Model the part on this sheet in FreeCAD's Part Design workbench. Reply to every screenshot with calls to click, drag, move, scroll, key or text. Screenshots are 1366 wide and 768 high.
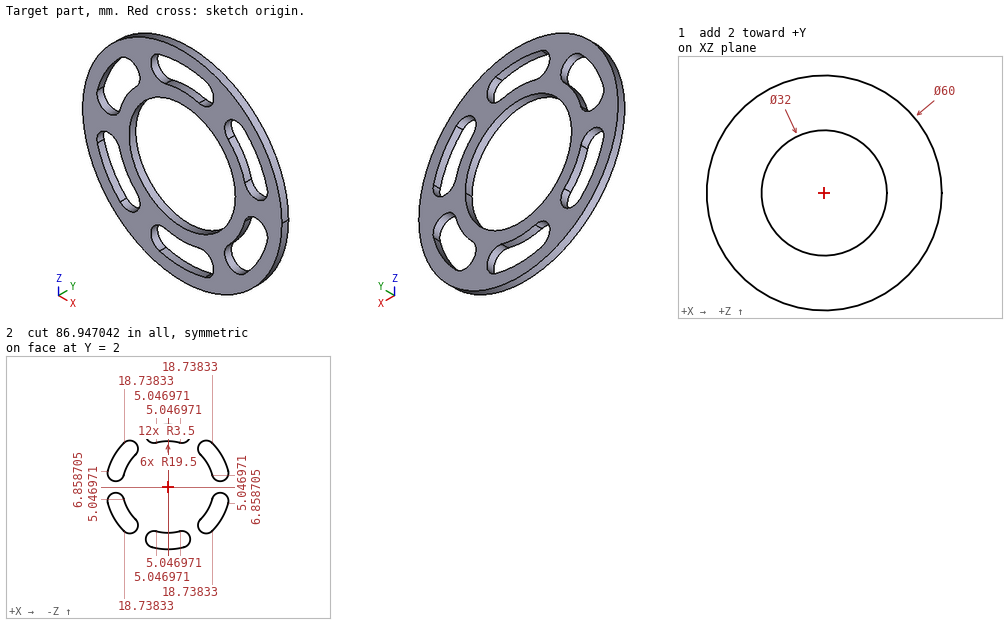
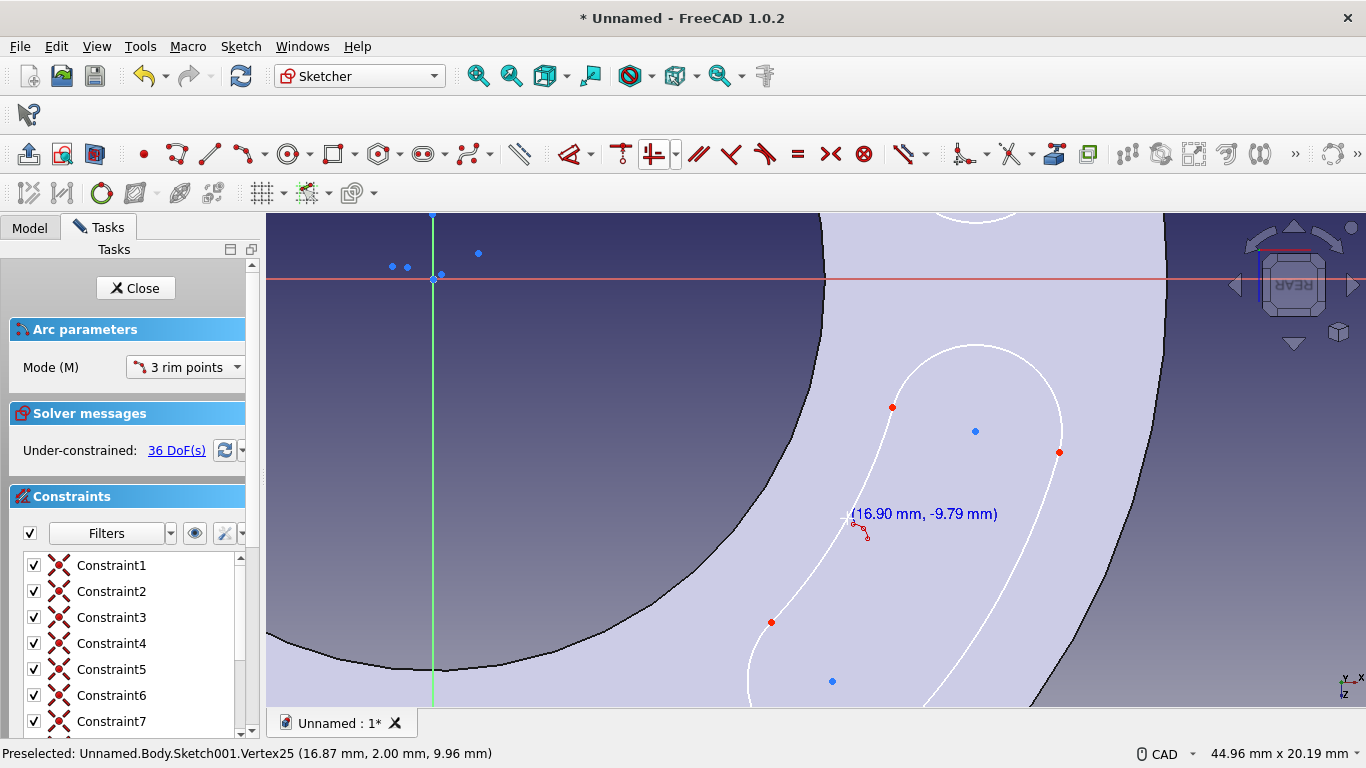
scroll(850, 519, down, 7)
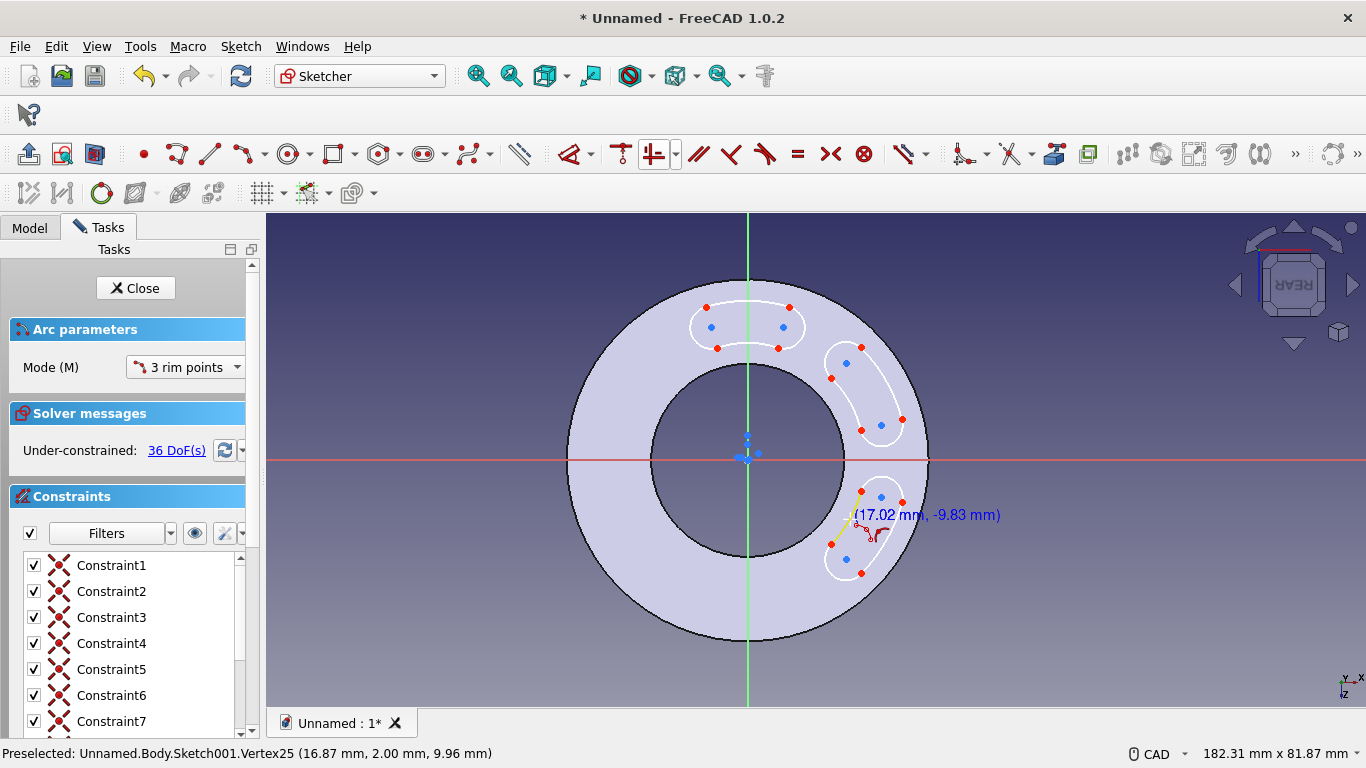
click(778, 574)
click(717, 574)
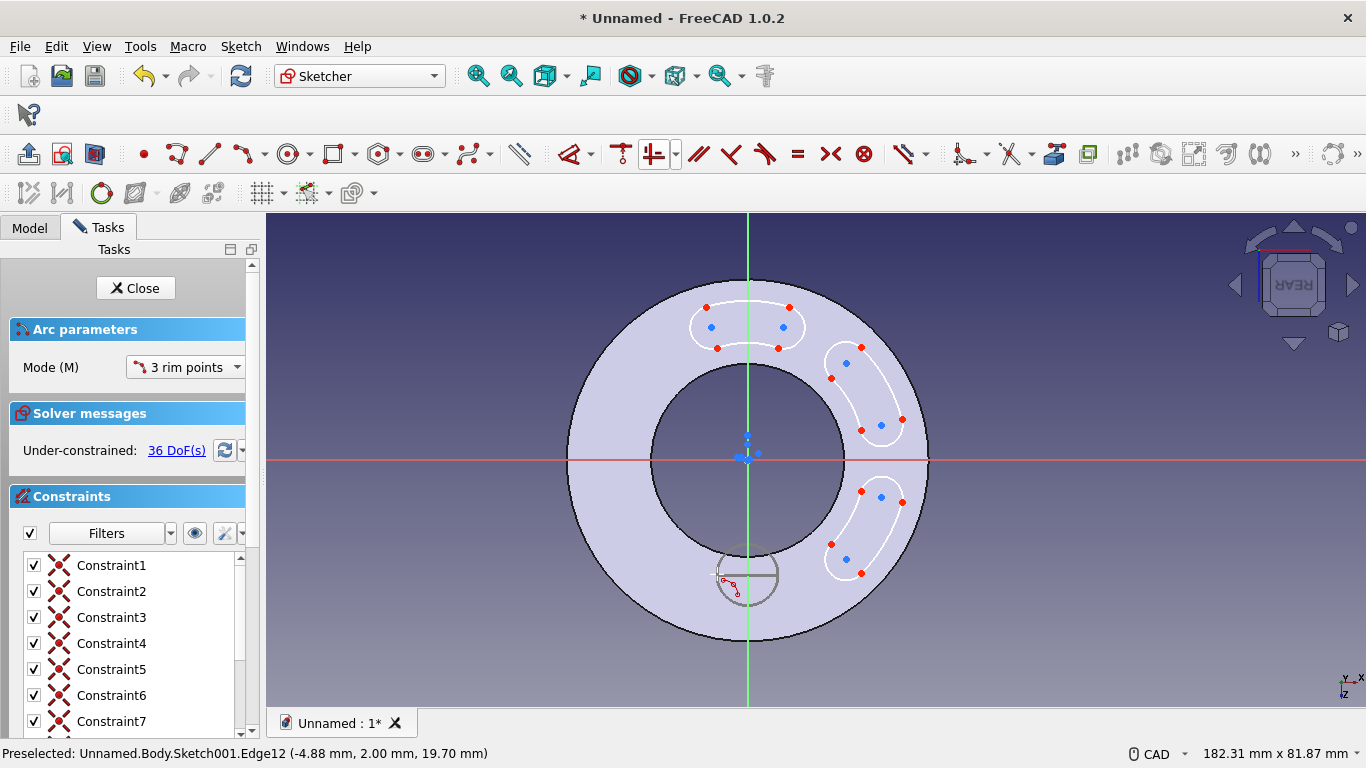
scroll(742, 578, up, 8)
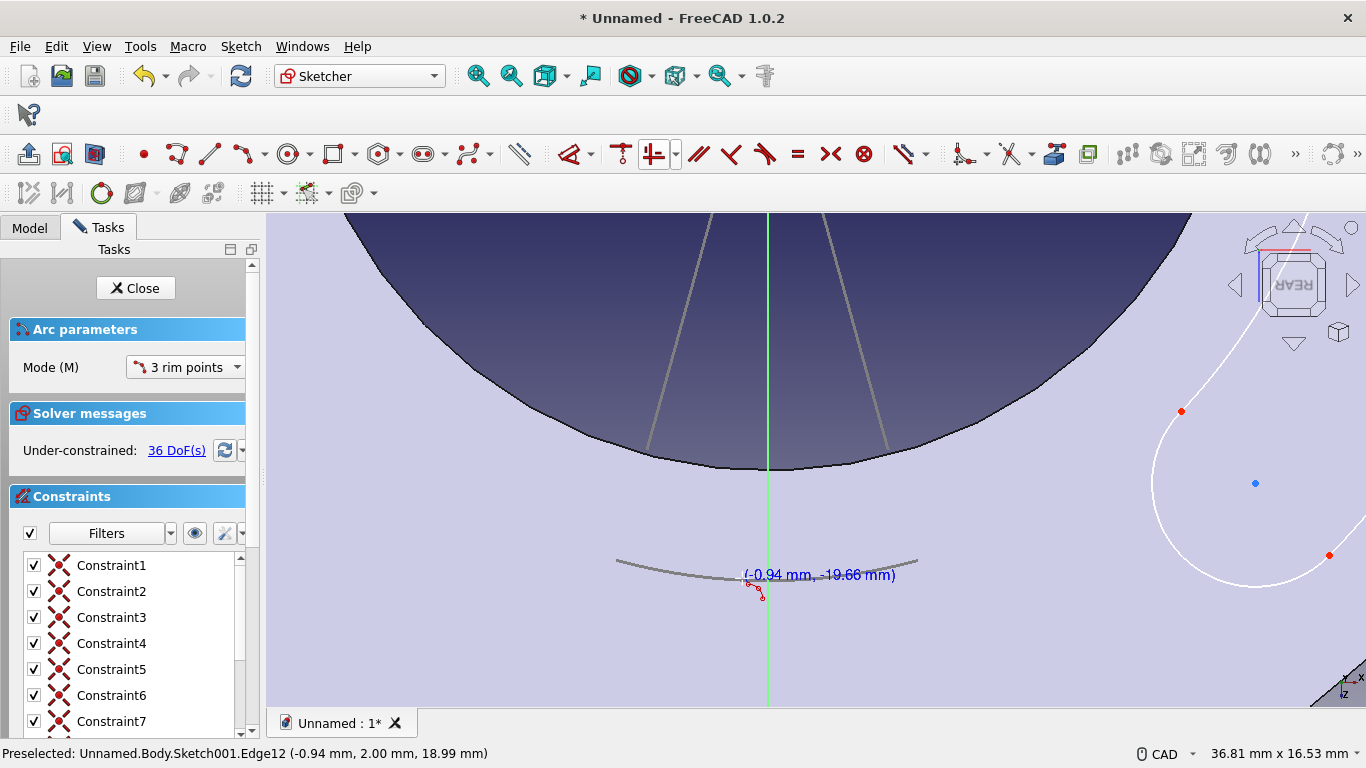
click(738, 575)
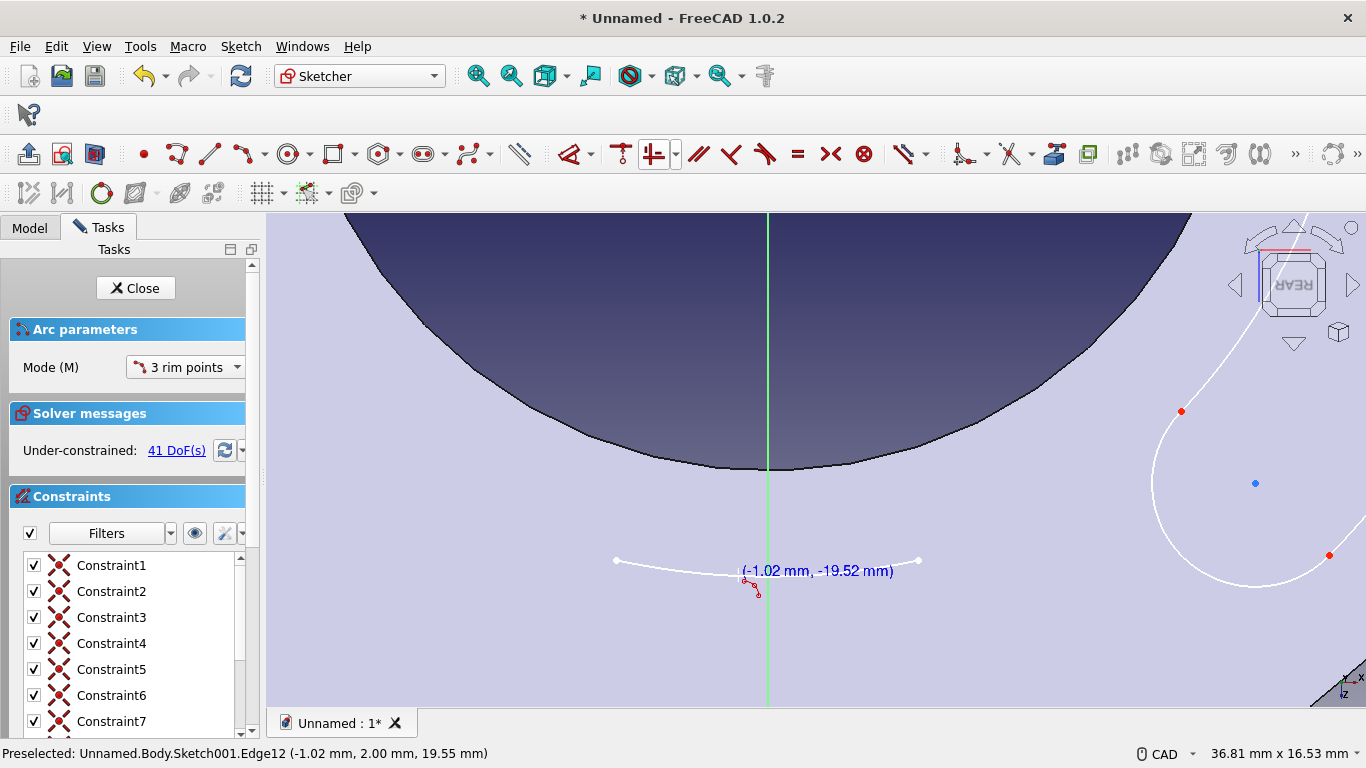
scroll(742, 578, down, 8)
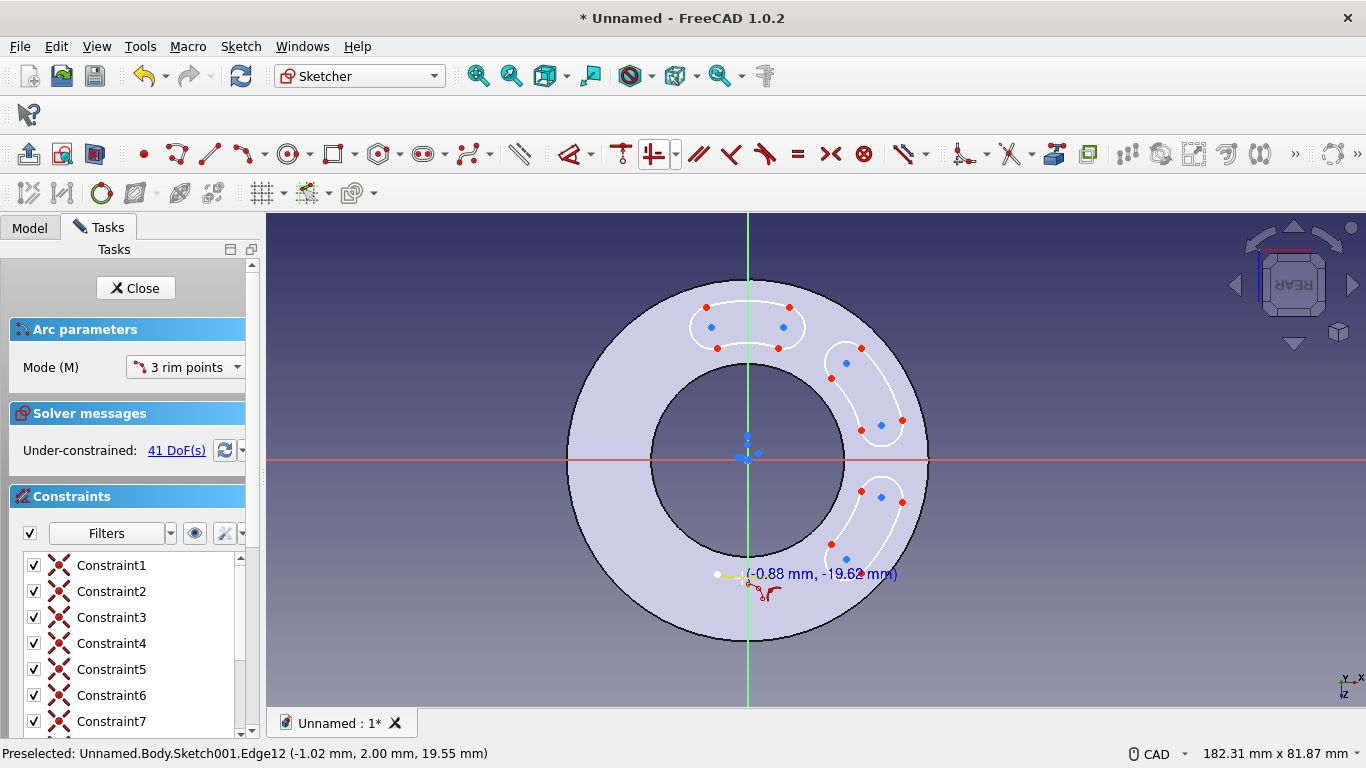
click(717, 575)
click(706, 615)
click(691, 589)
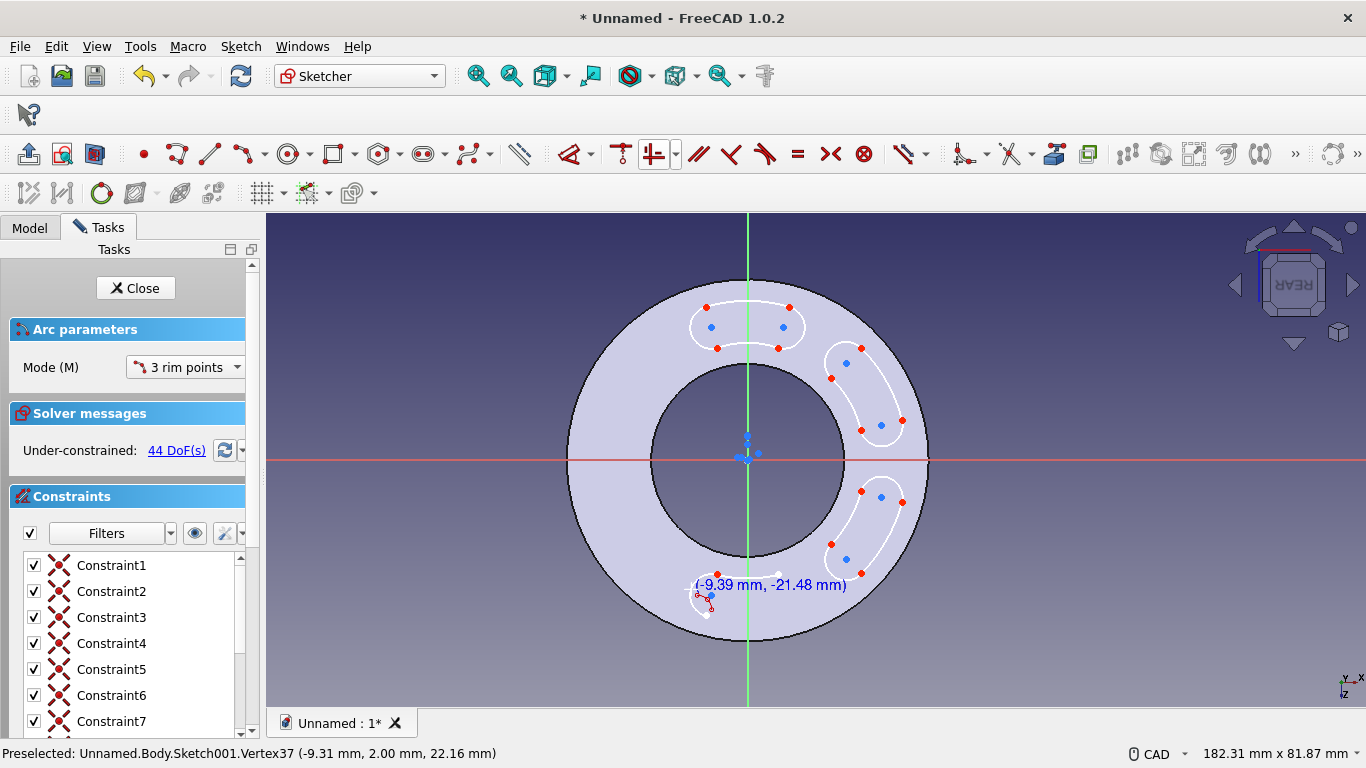
click(706, 616)
click(789, 615)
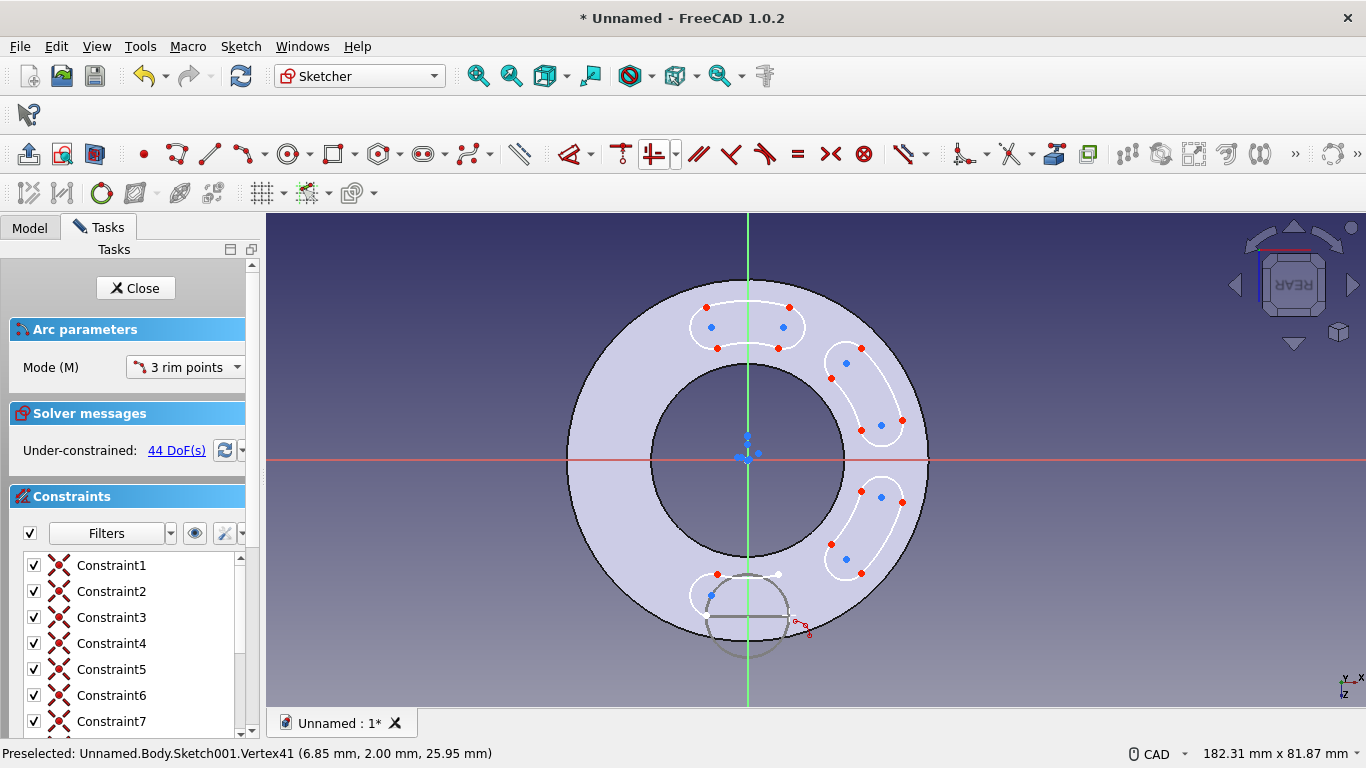
scroll(739, 620, up, 6)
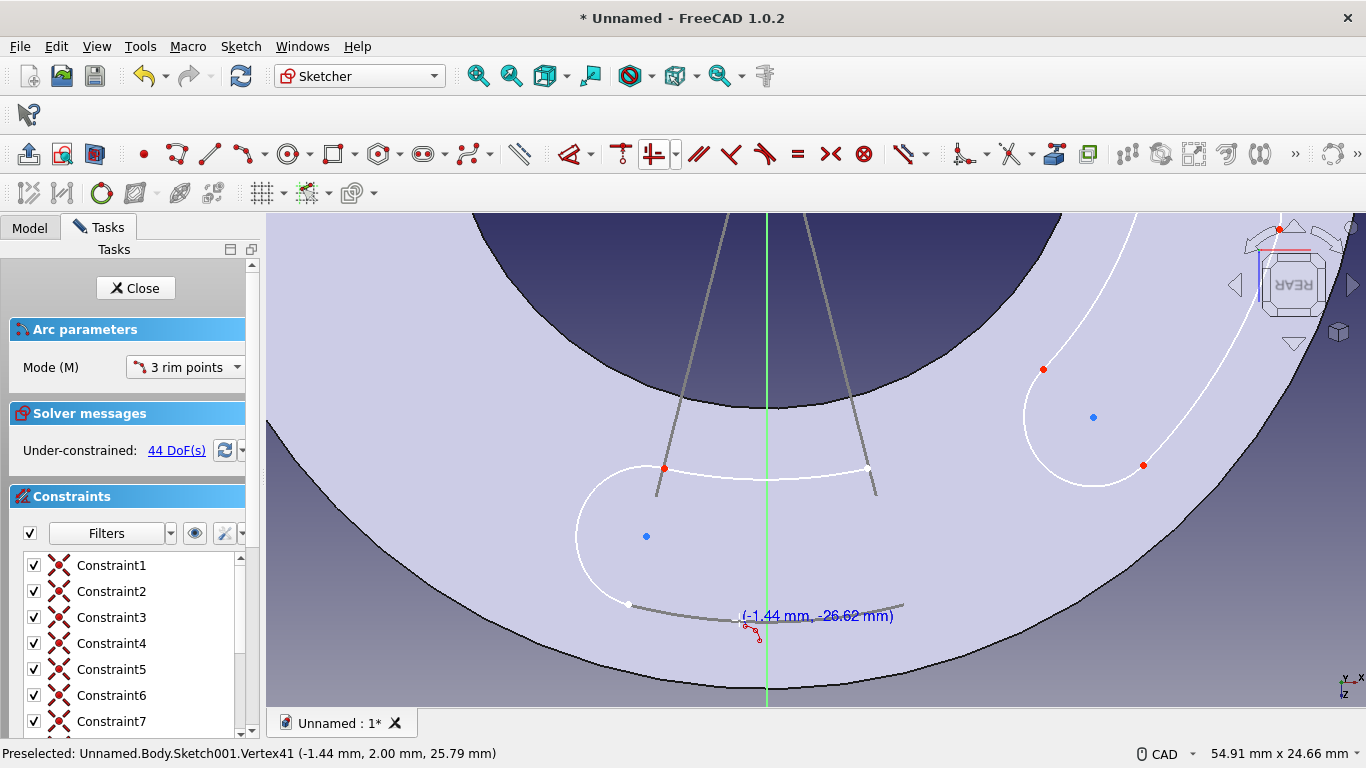
click(739, 618)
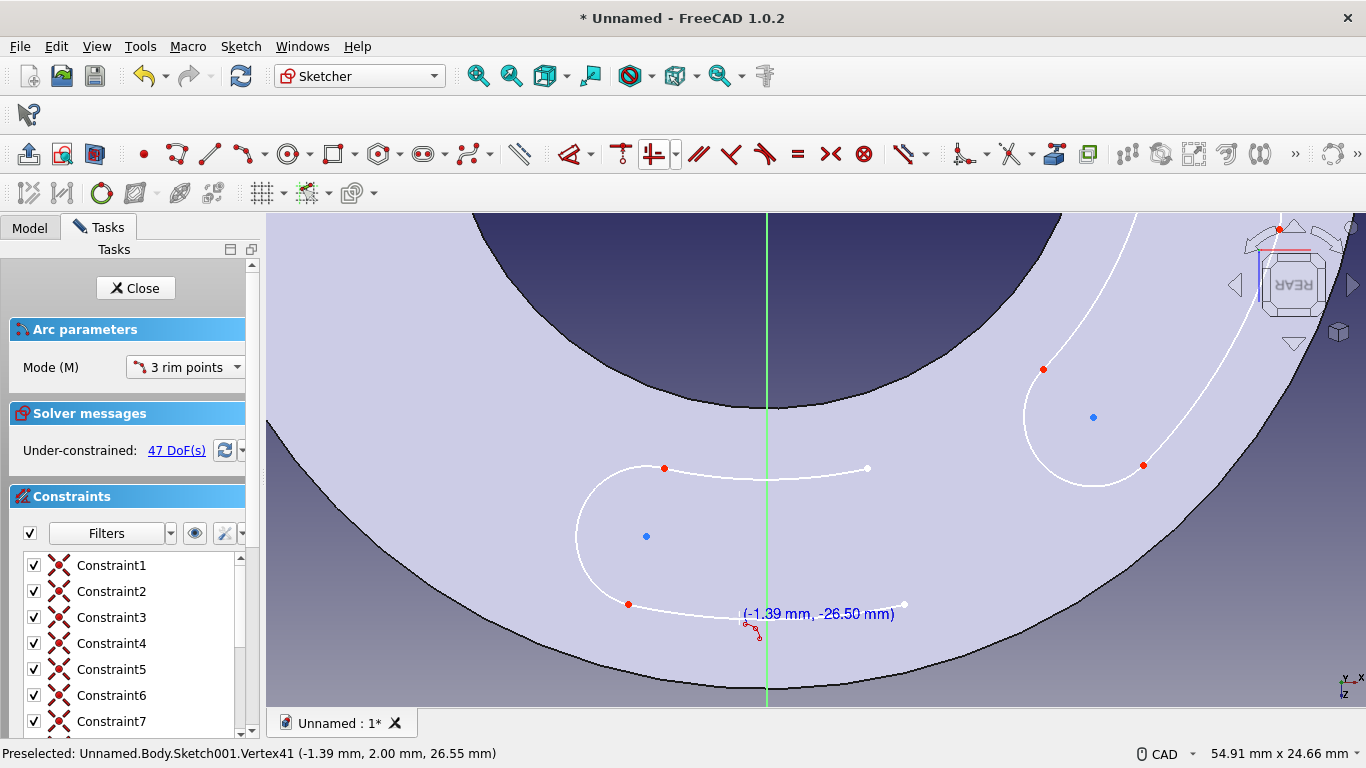
scroll(739, 620, down, 6)